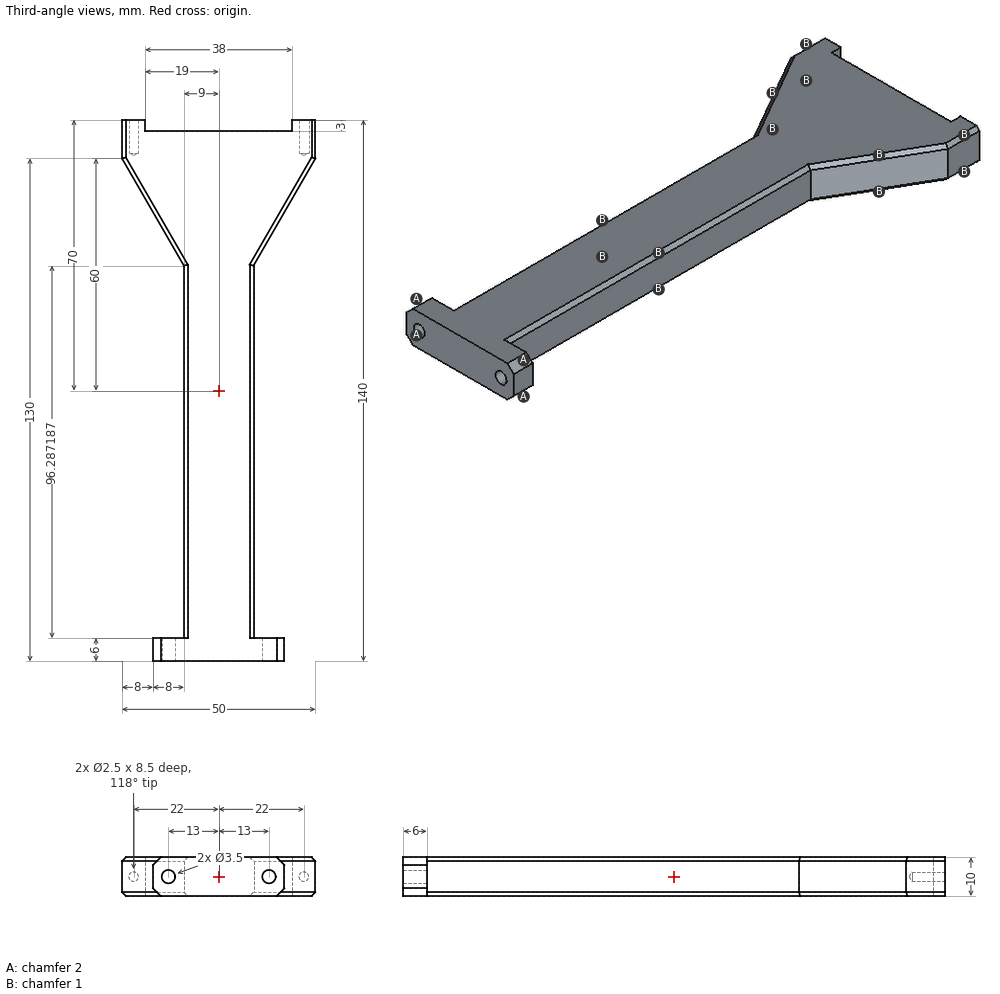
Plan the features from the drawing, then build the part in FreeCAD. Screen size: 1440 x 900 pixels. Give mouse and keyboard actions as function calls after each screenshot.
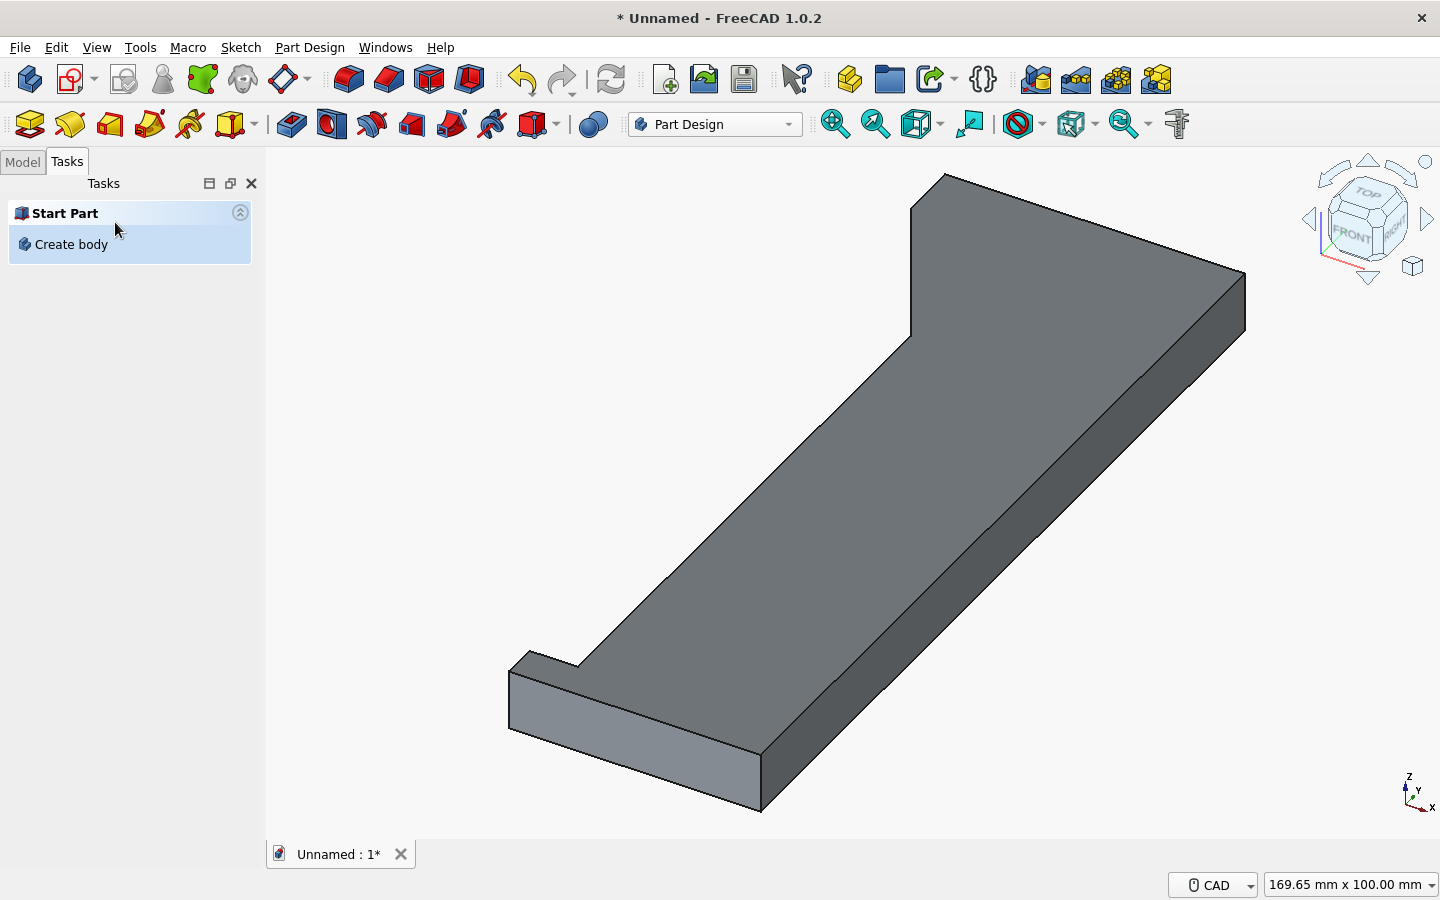
click(23, 161)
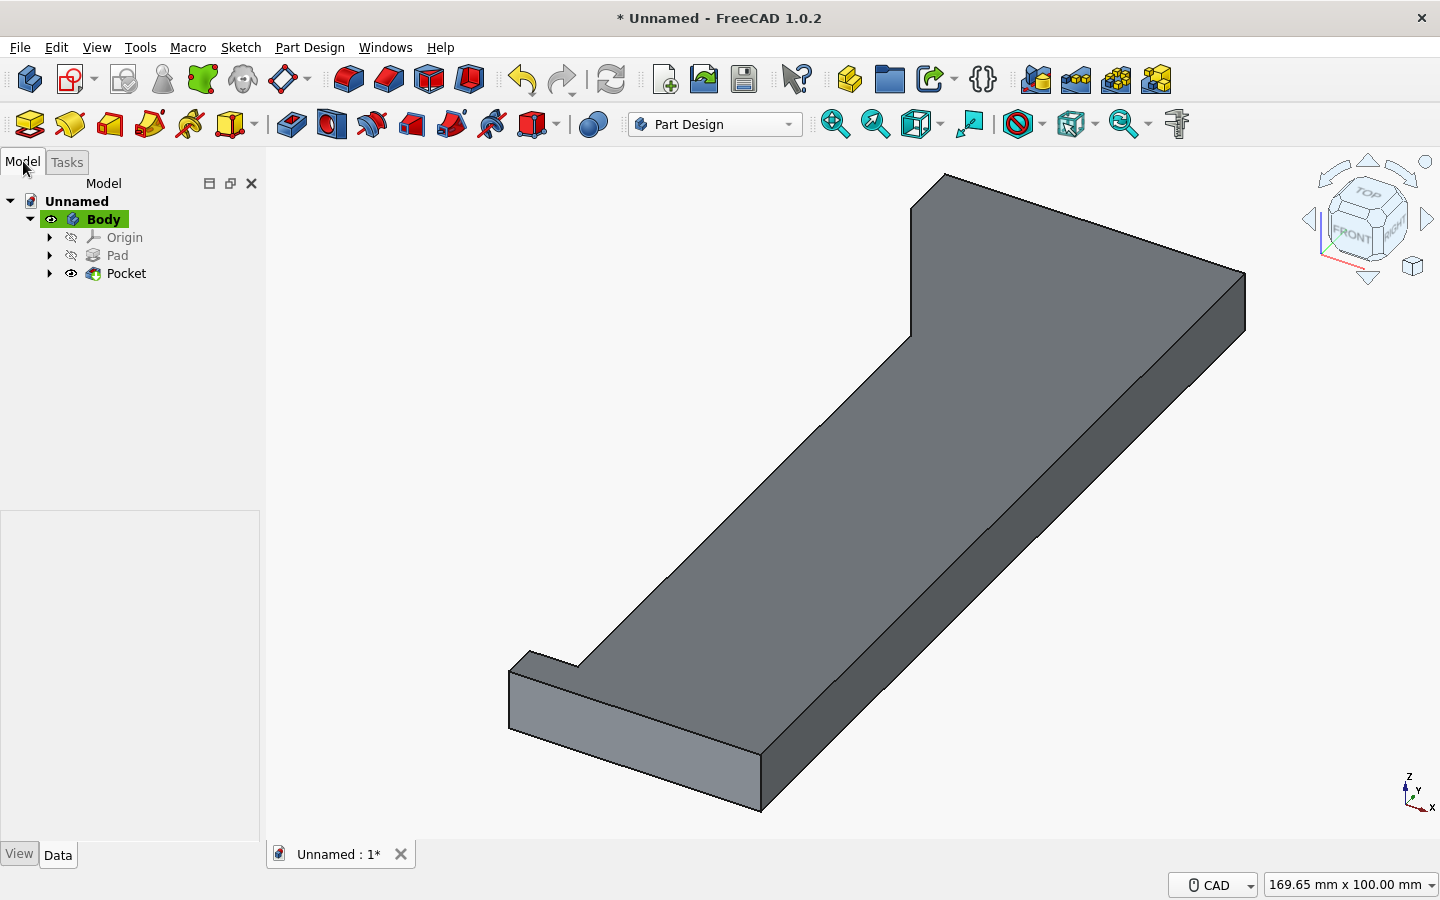
click(116, 273)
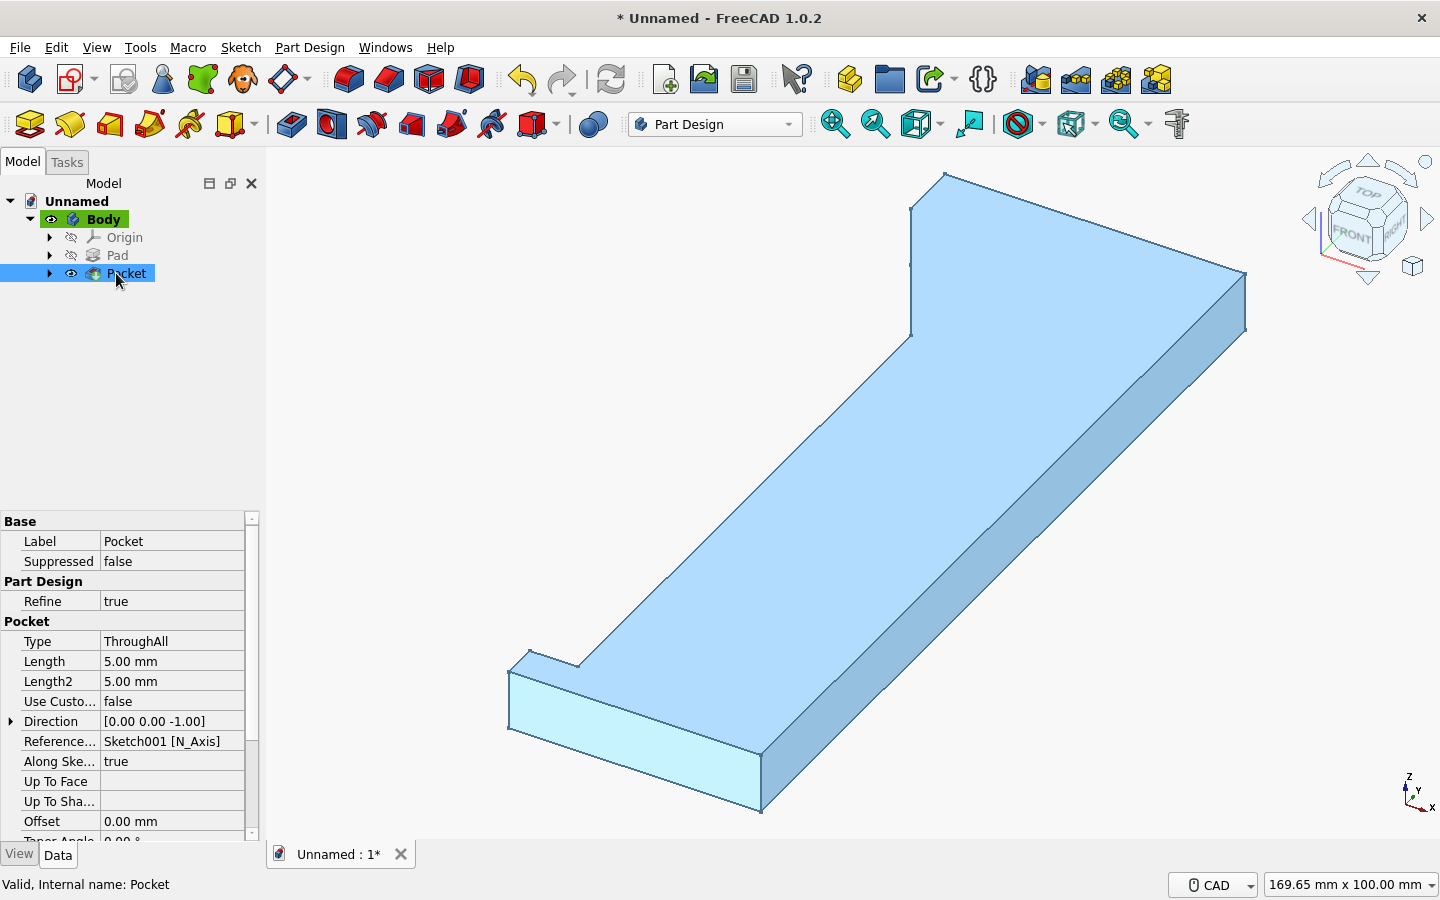
click(1036, 80)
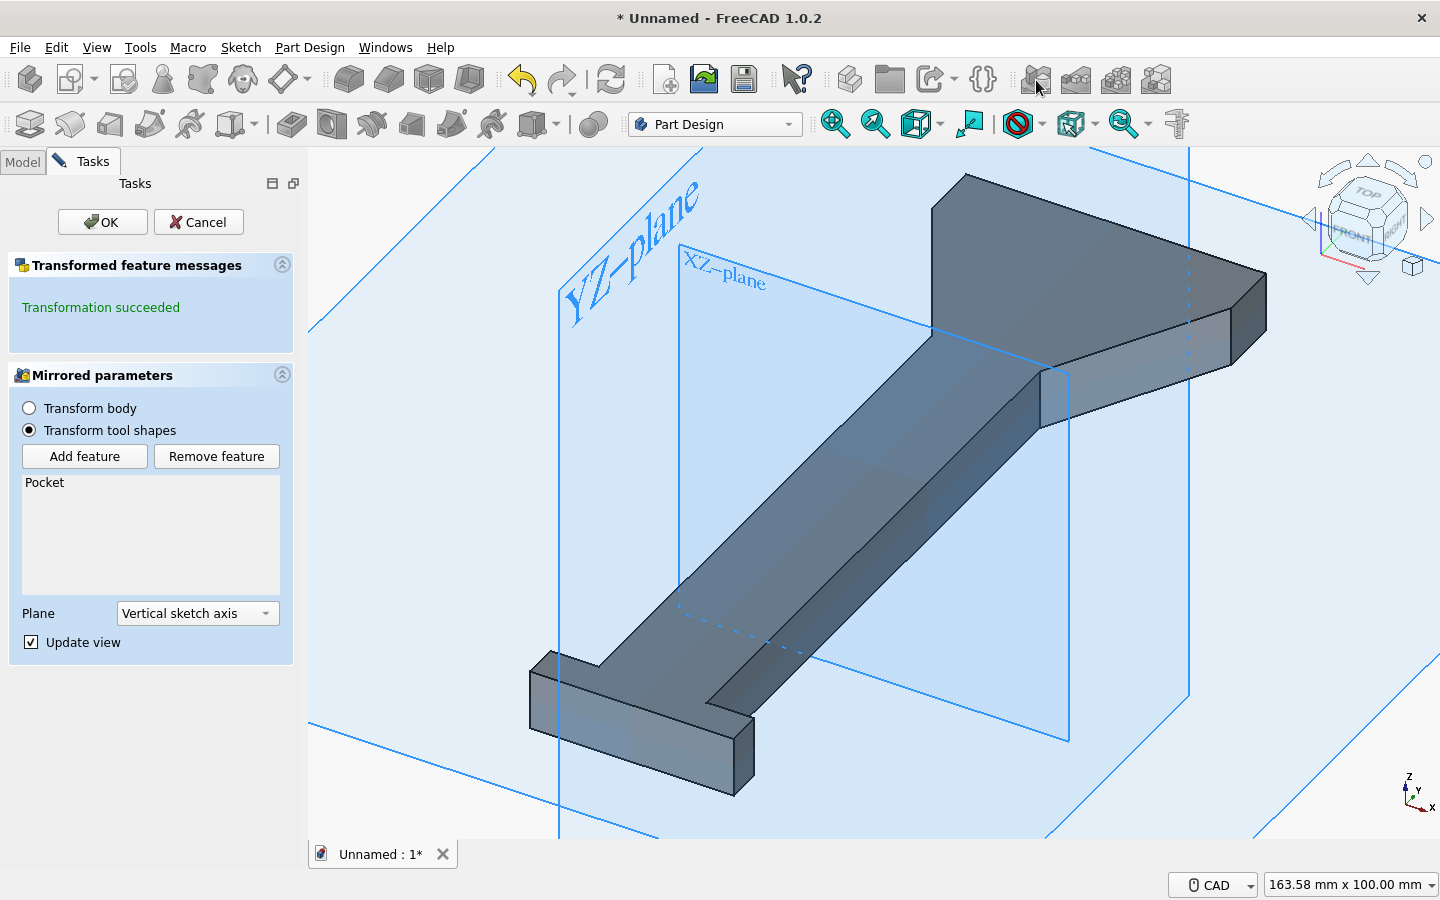
click(198, 614)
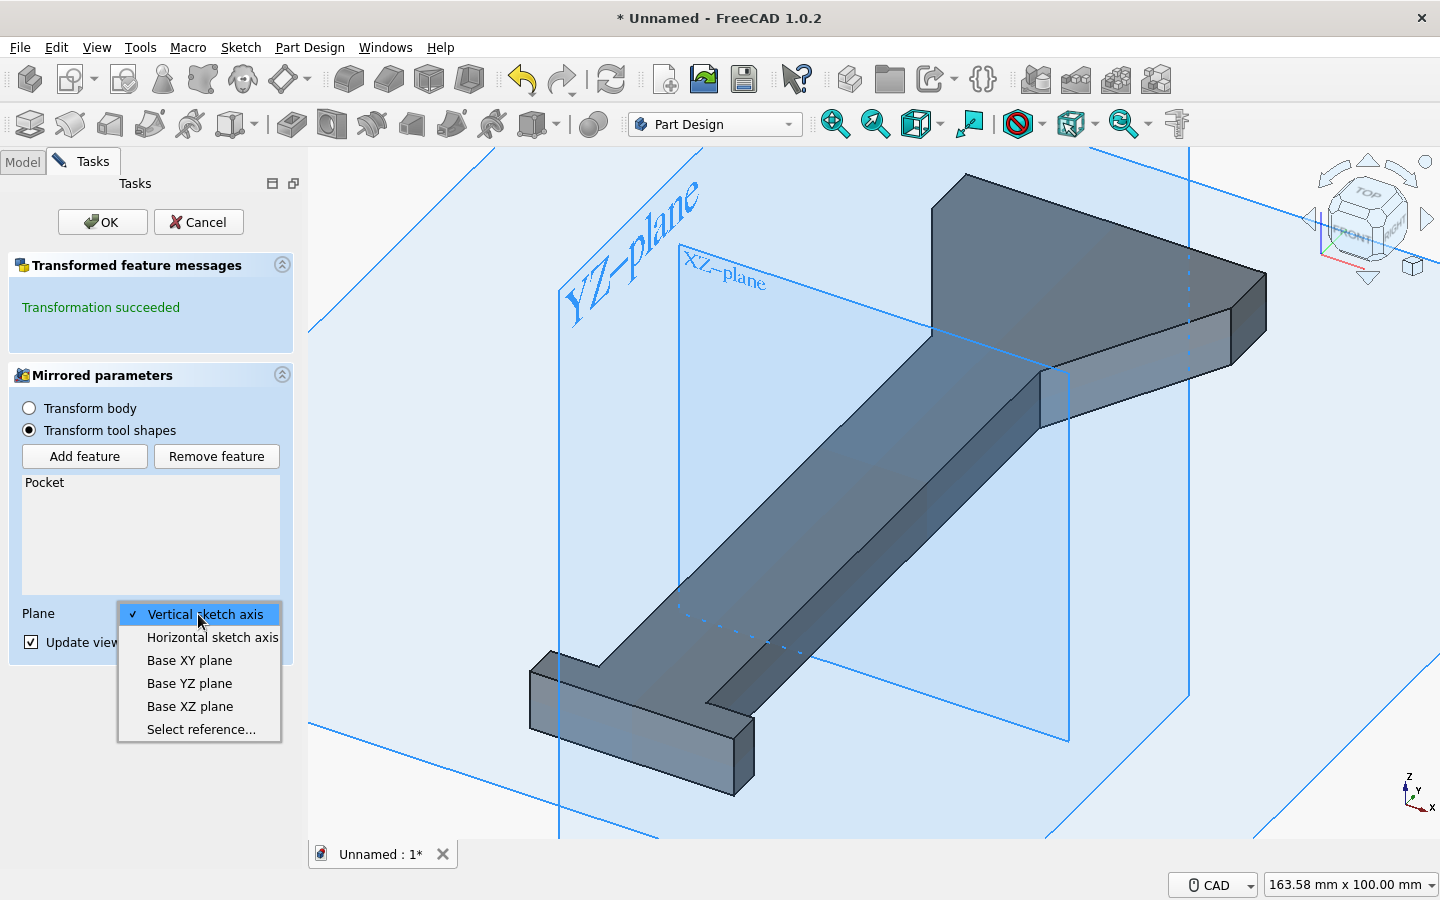
click(198, 684)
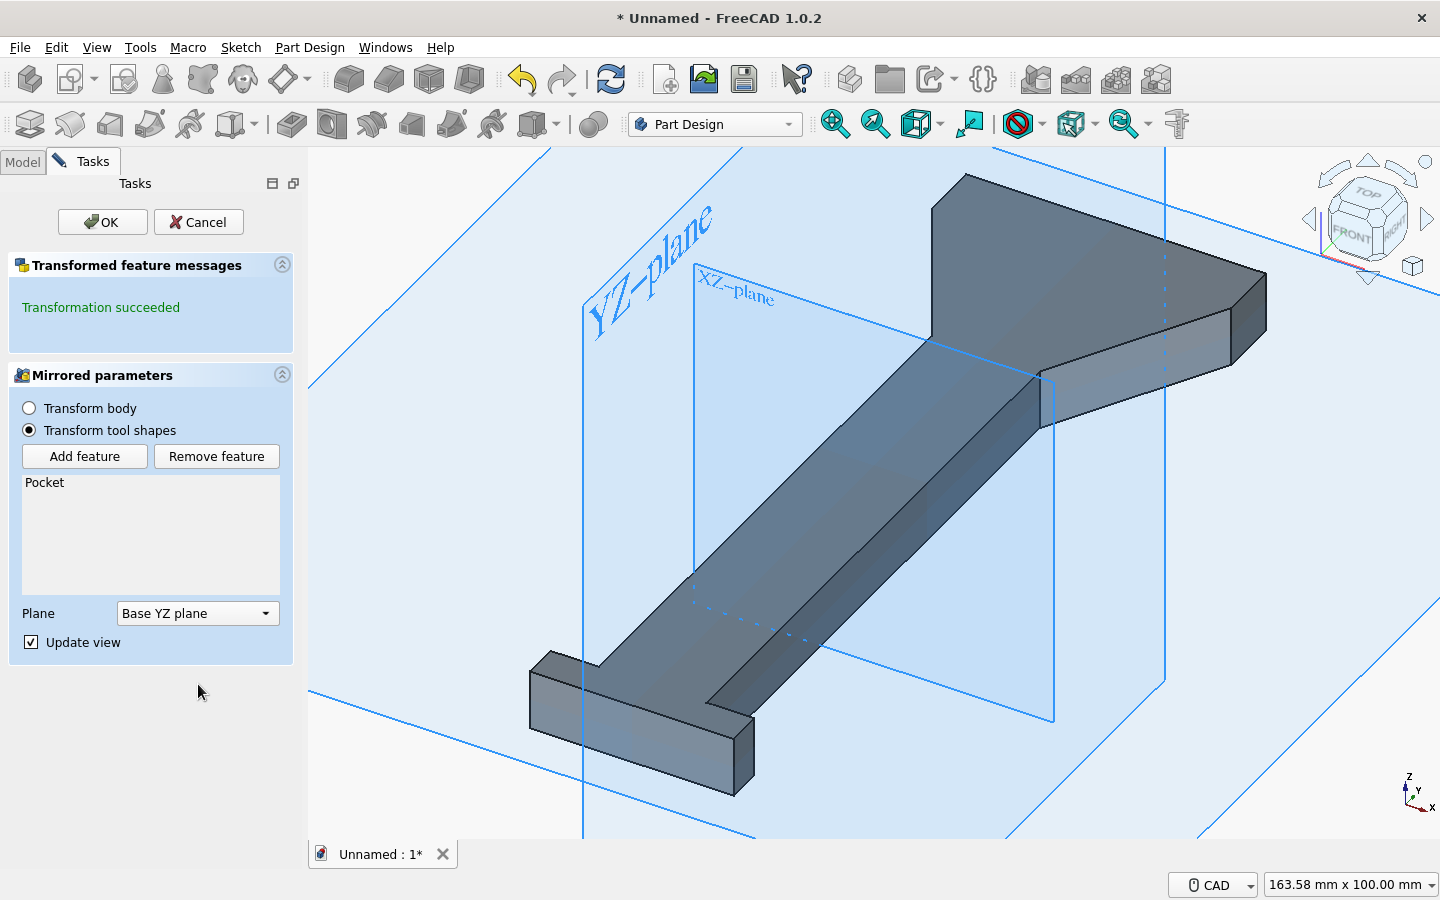
click(103, 222)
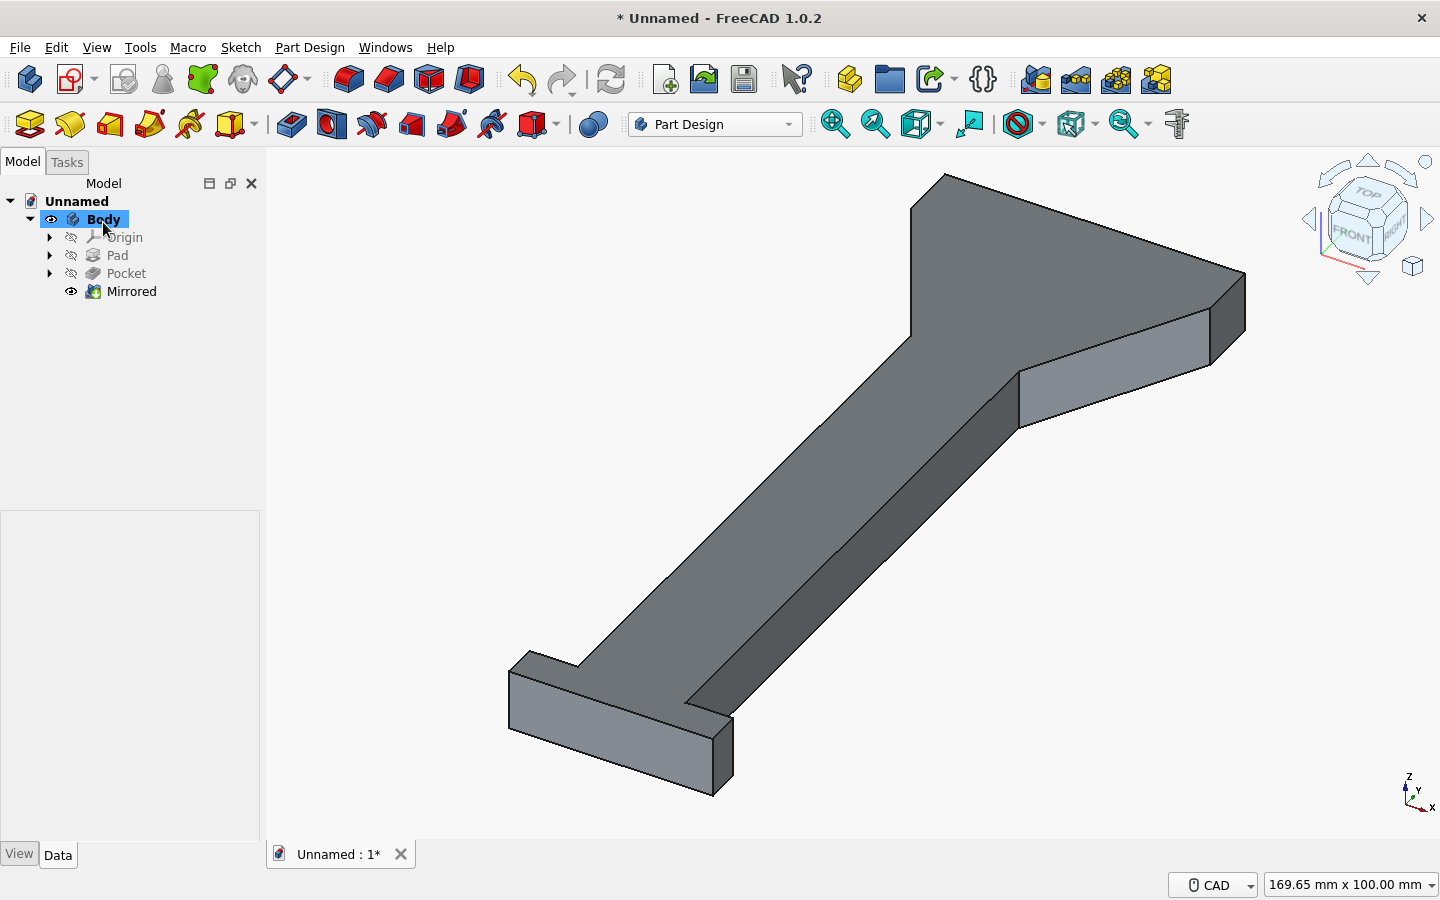
click(991, 326)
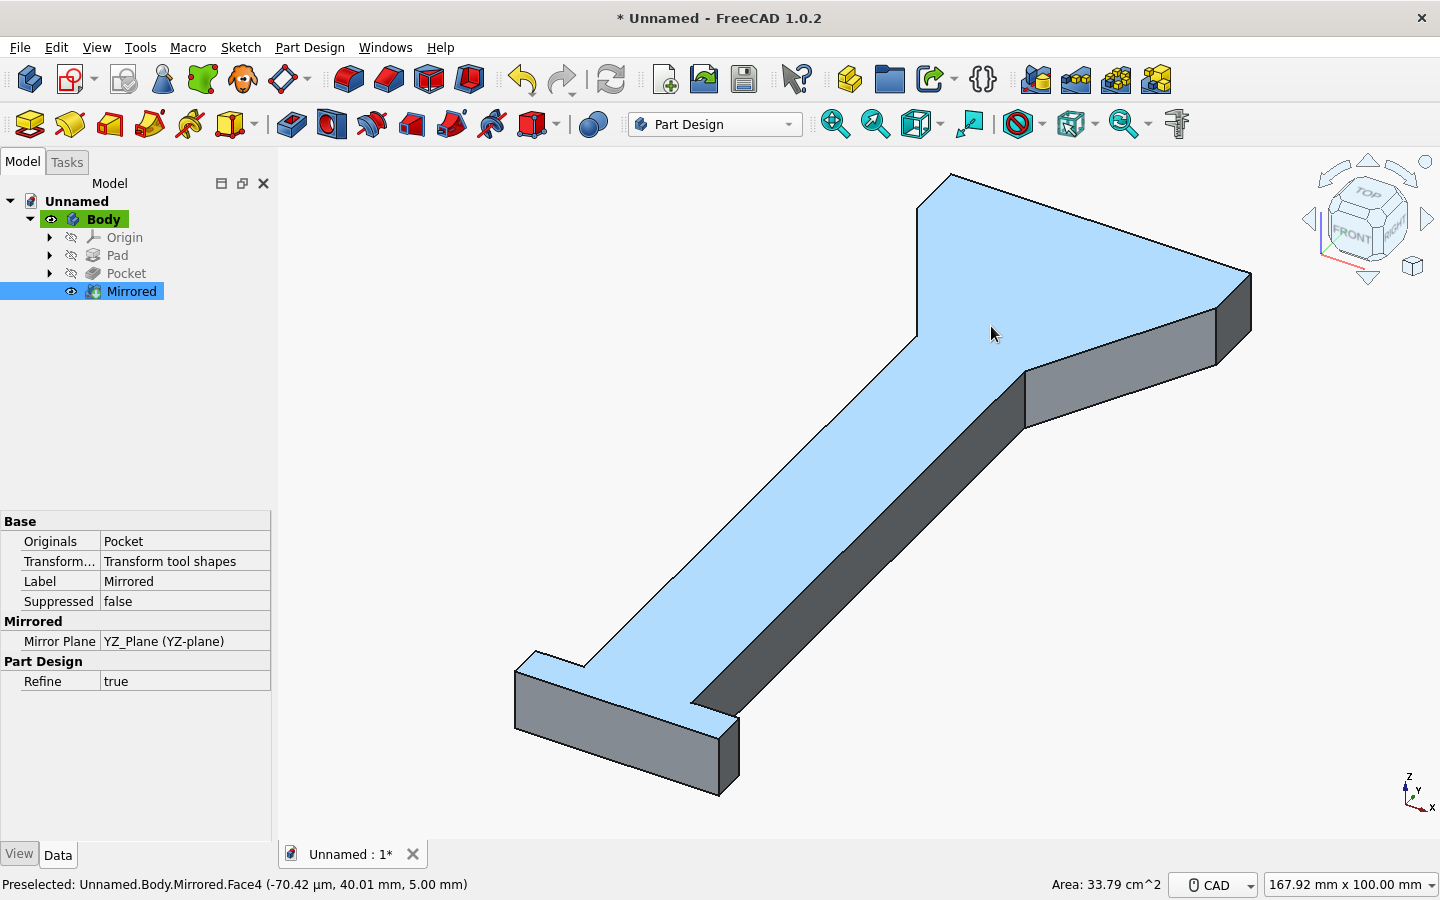
click(70, 80)